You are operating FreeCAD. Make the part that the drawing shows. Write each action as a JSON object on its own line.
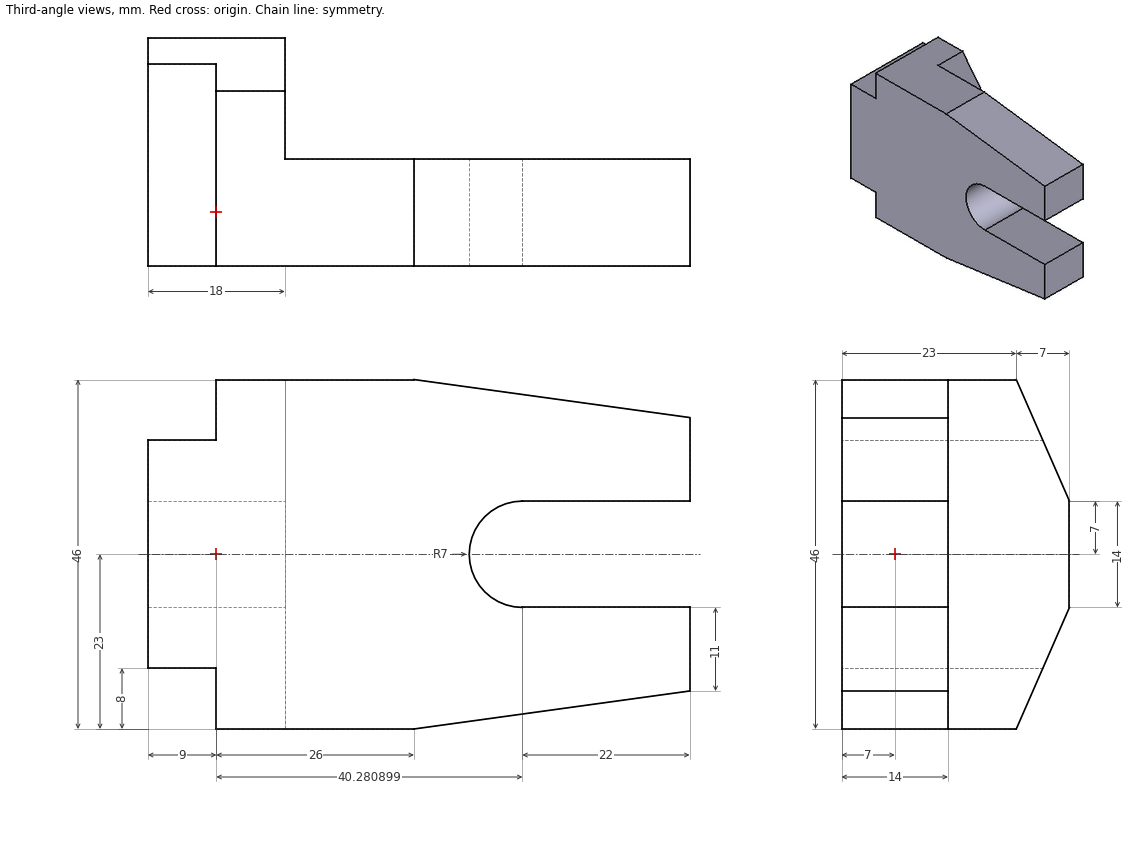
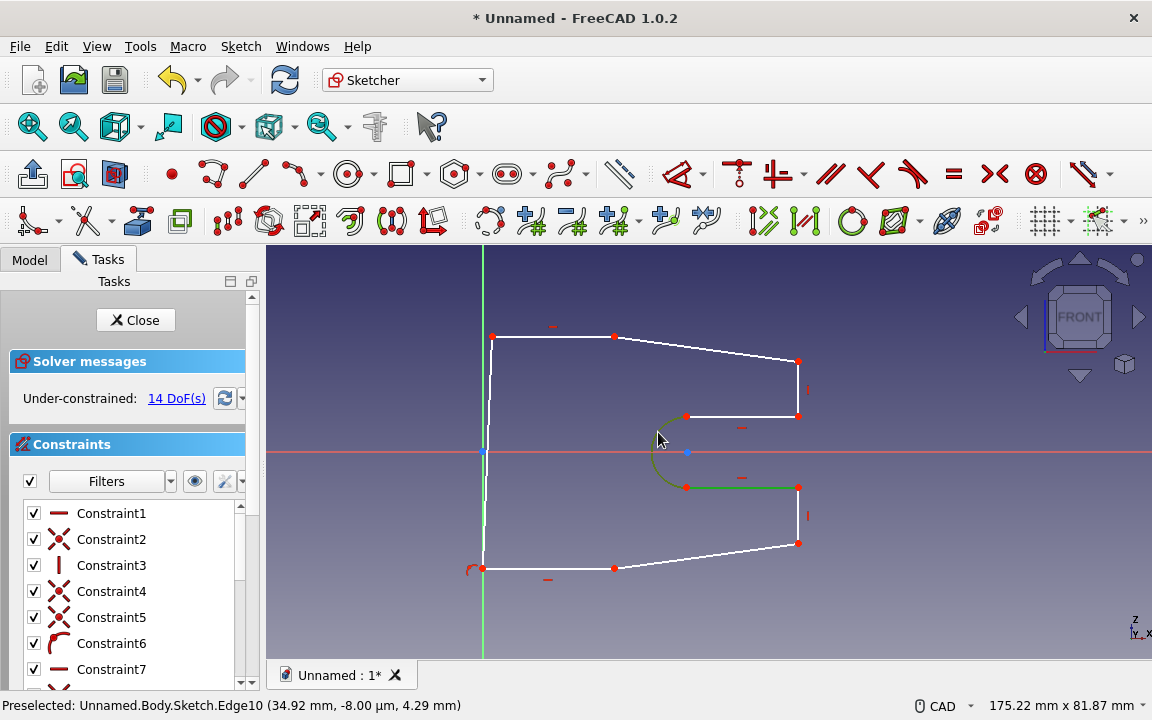
{"action": "key", "text": "t"}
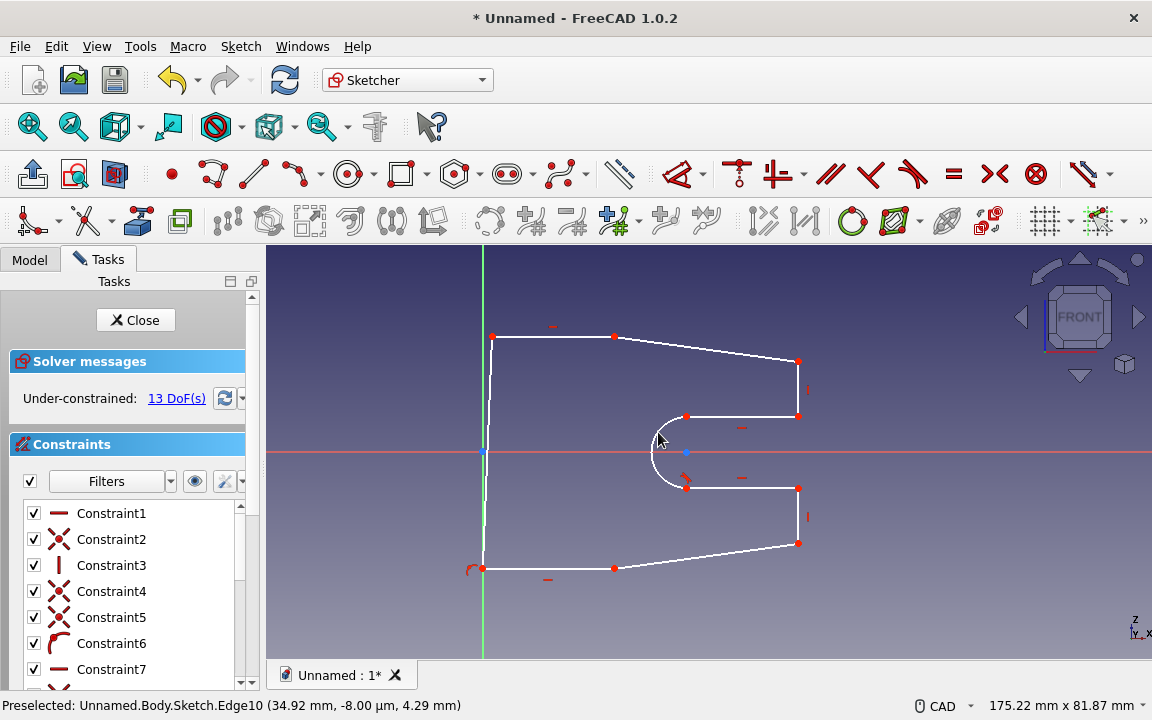
{"action": "left_click", "coordinate": [764, 417]}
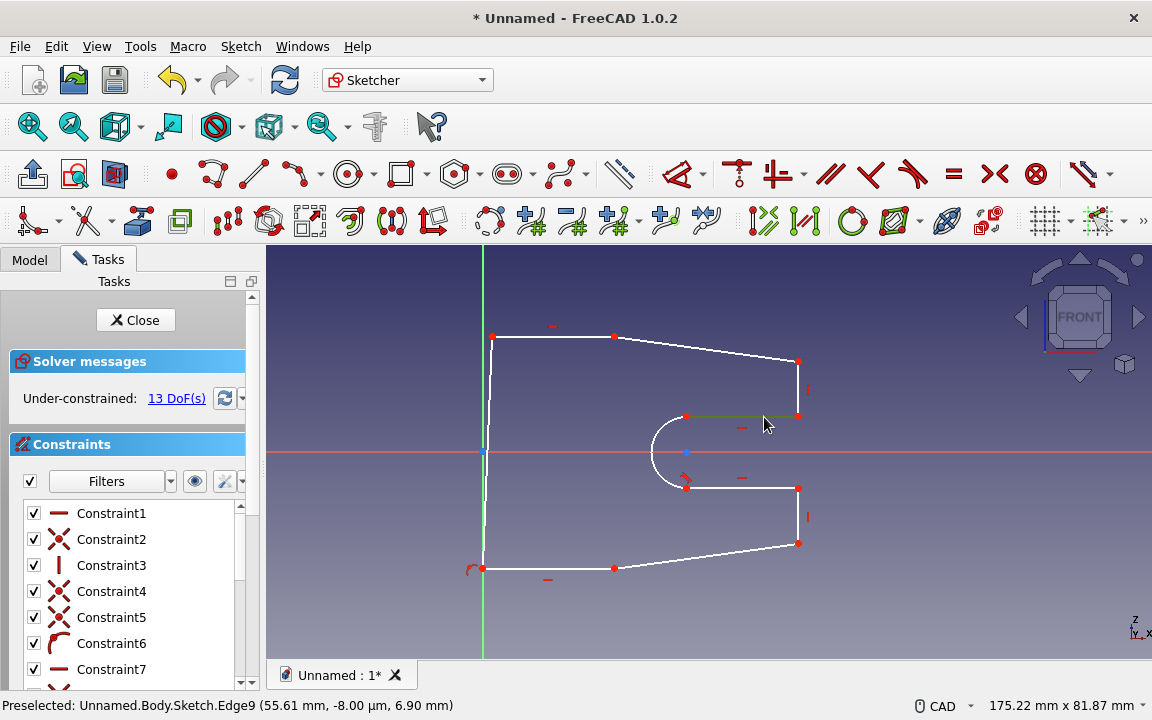
{"action": "left_click", "coordinate": [658, 432]}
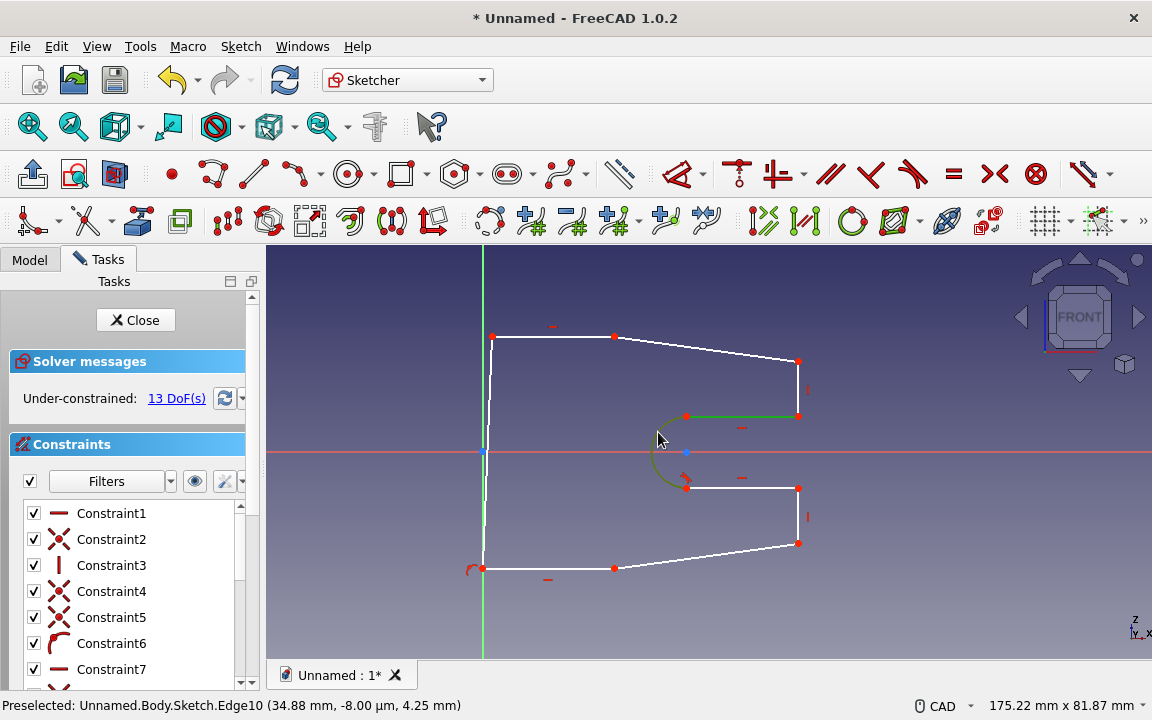
{"action": "key", "text": "t"}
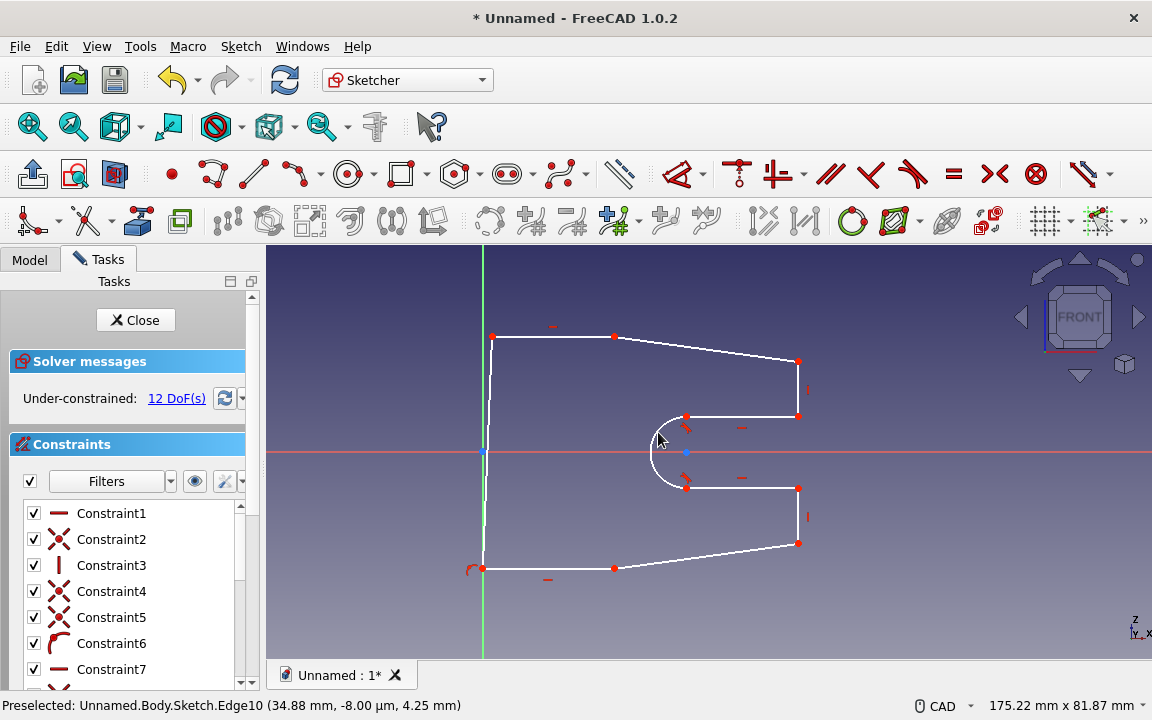
{"action": "left_click", "coordinate": [486, 499]}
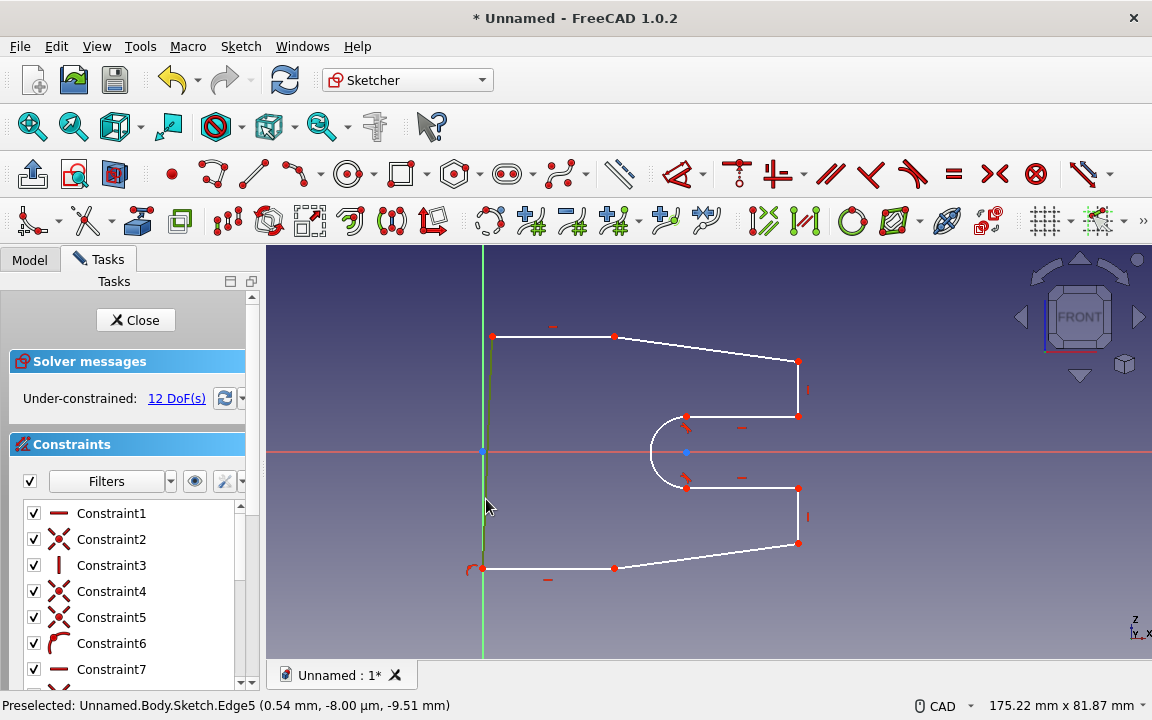
{"action": "key", "text": "v"}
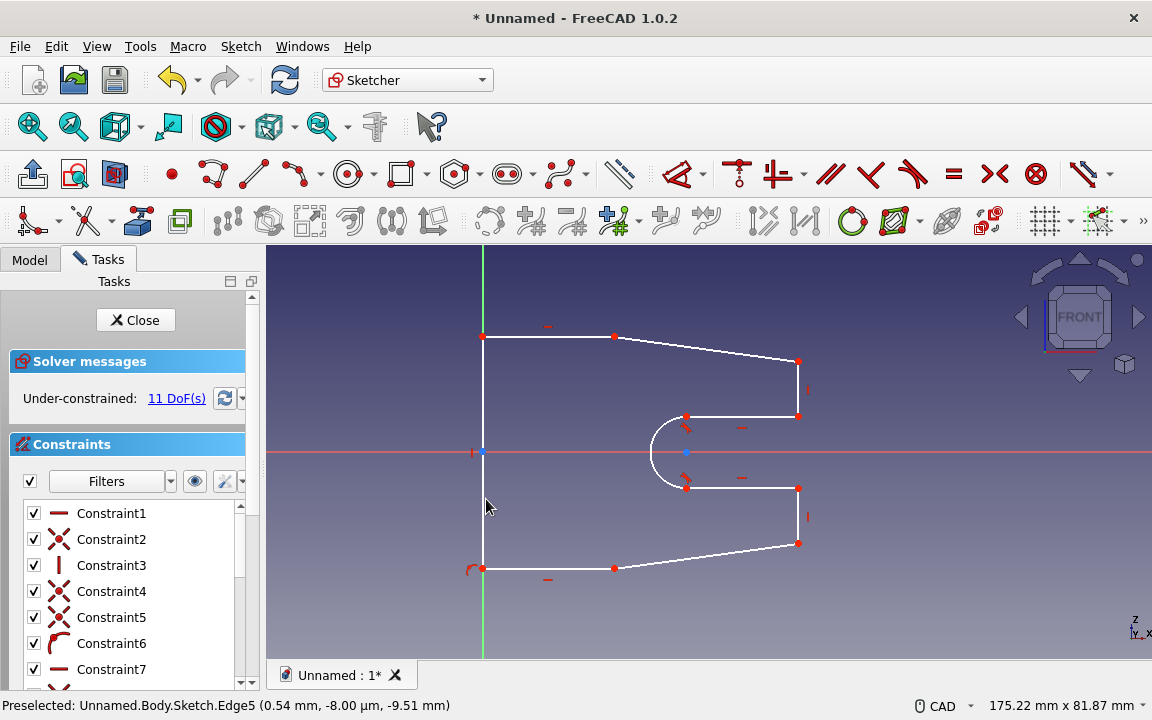
{"action": "left_click", "coordinate": [686, 452]}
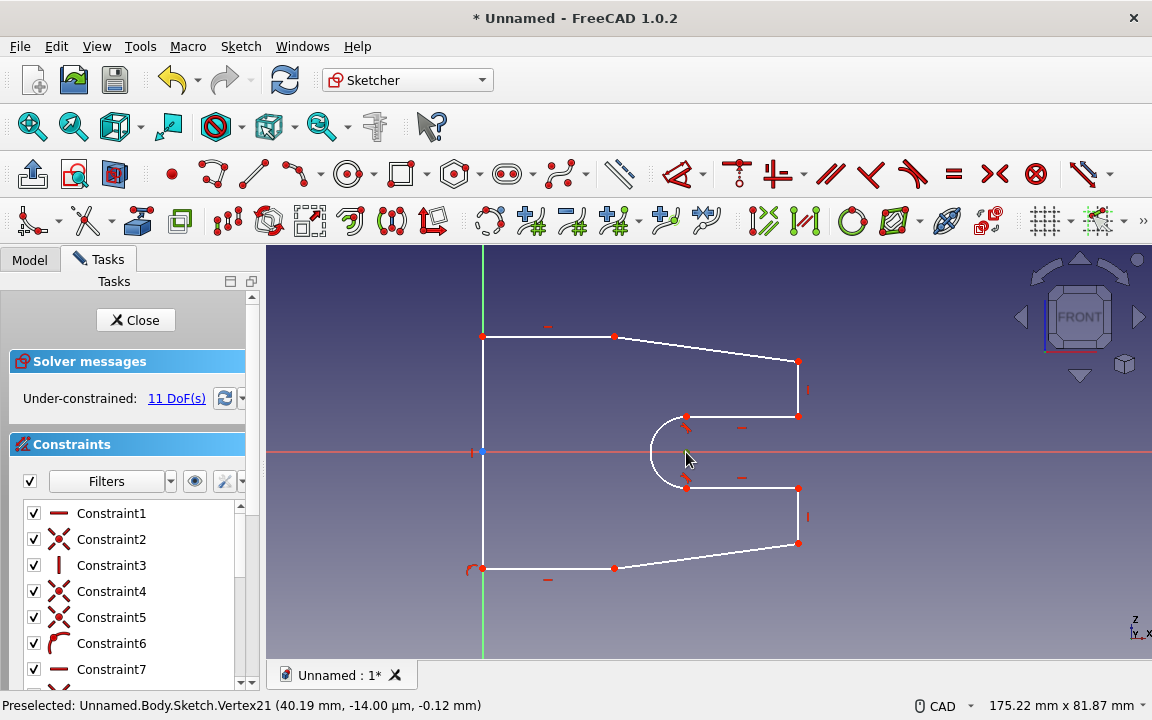
{"action": "left_click", "coordinate": [344, 452]}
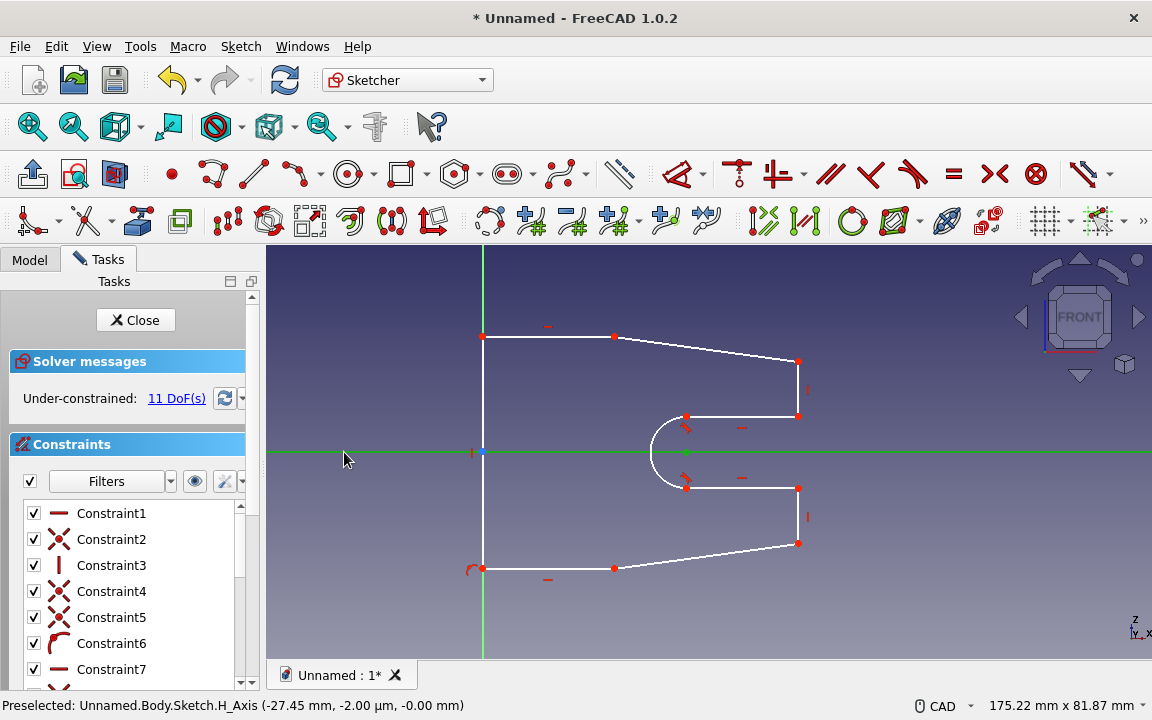
{"action": "key", "text": "c"}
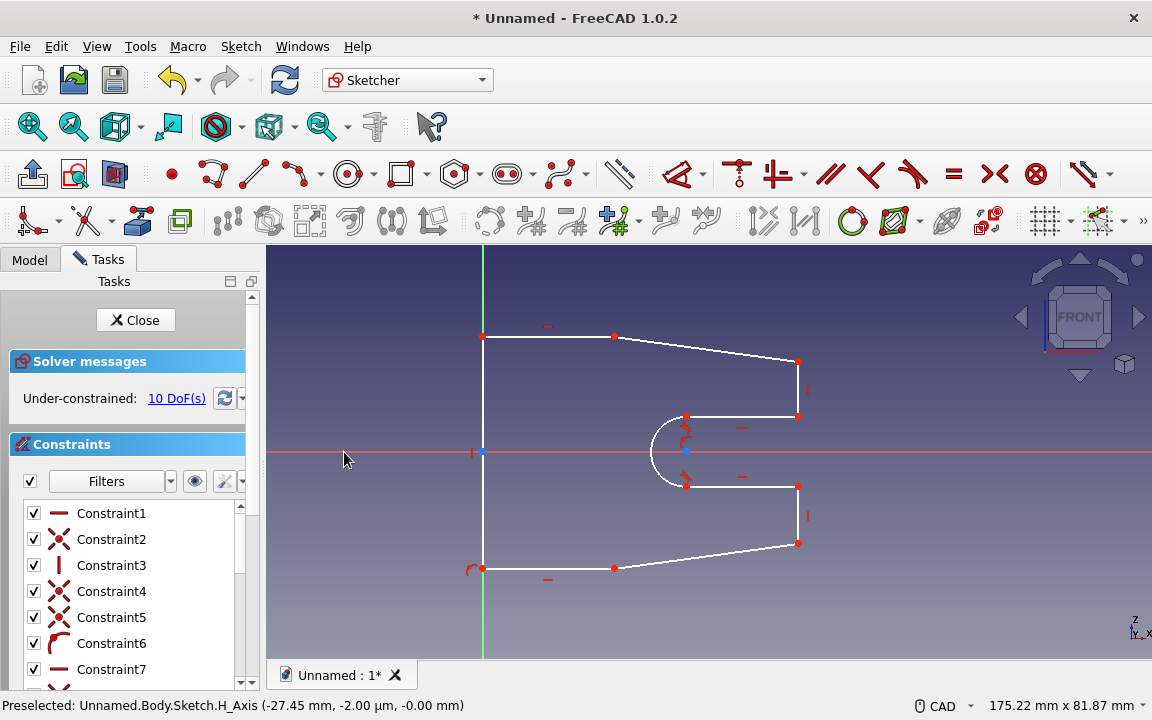
{"action": "left_click", "coordinate": [614, 569]}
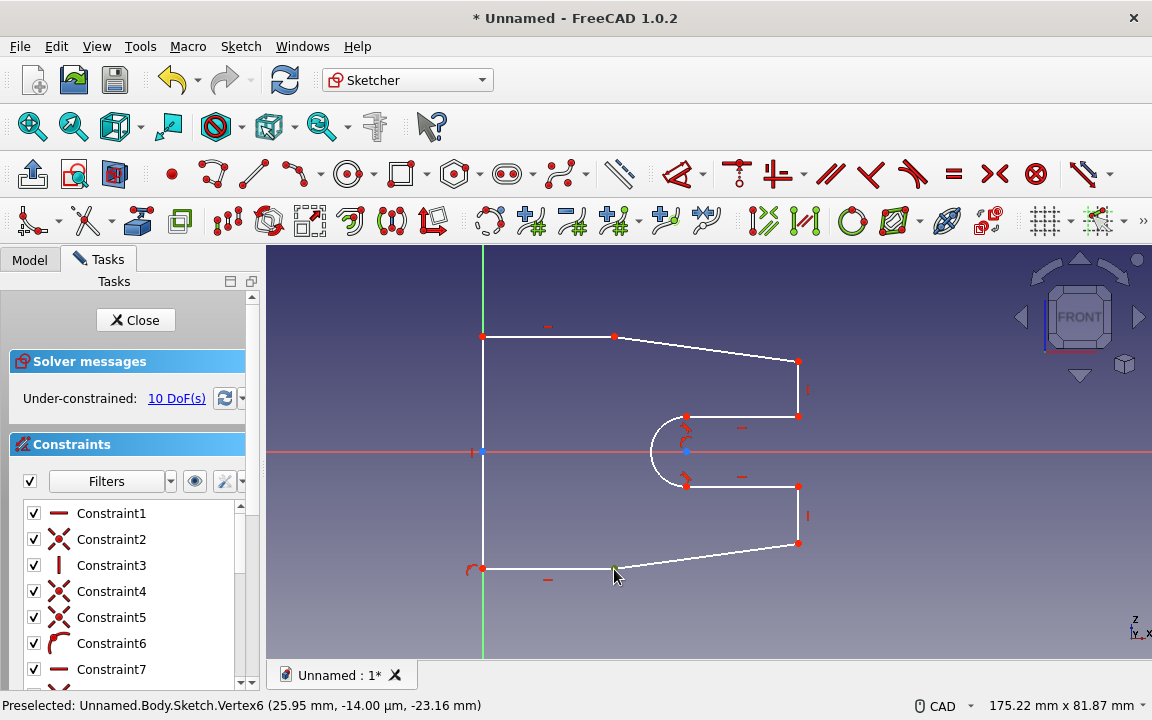
{"action": "left_click", "coordinate": [614, 337]}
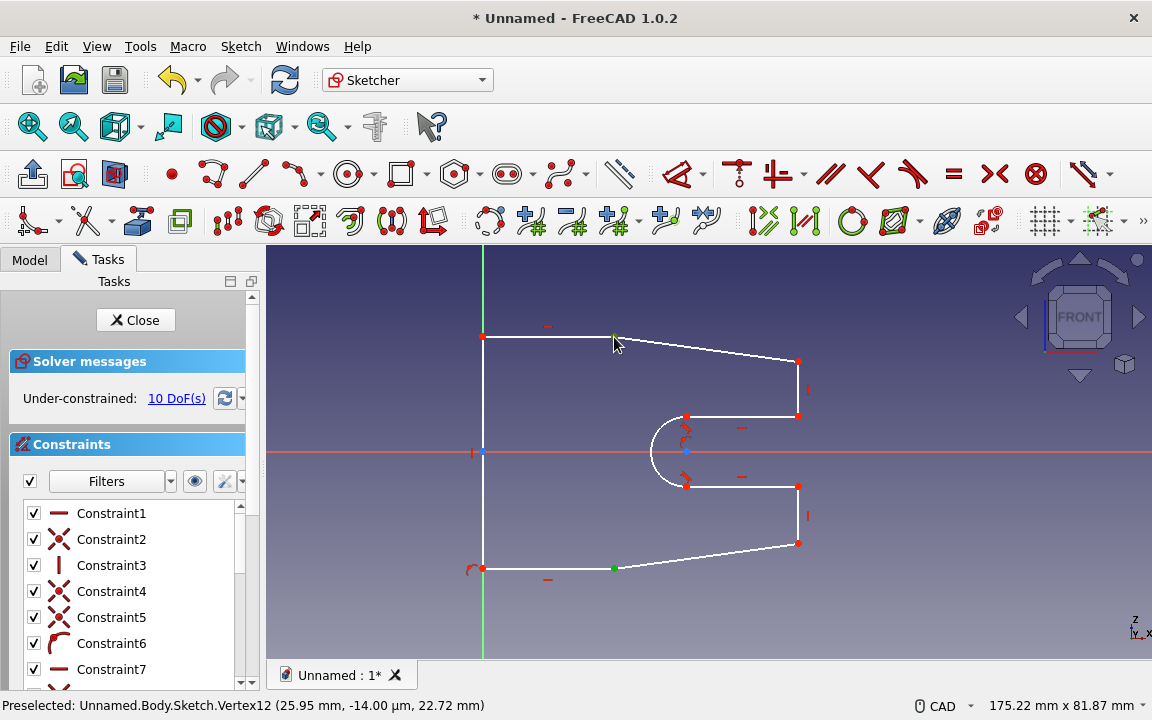
{"action": "left_click", "coordinate": [344, 452]}